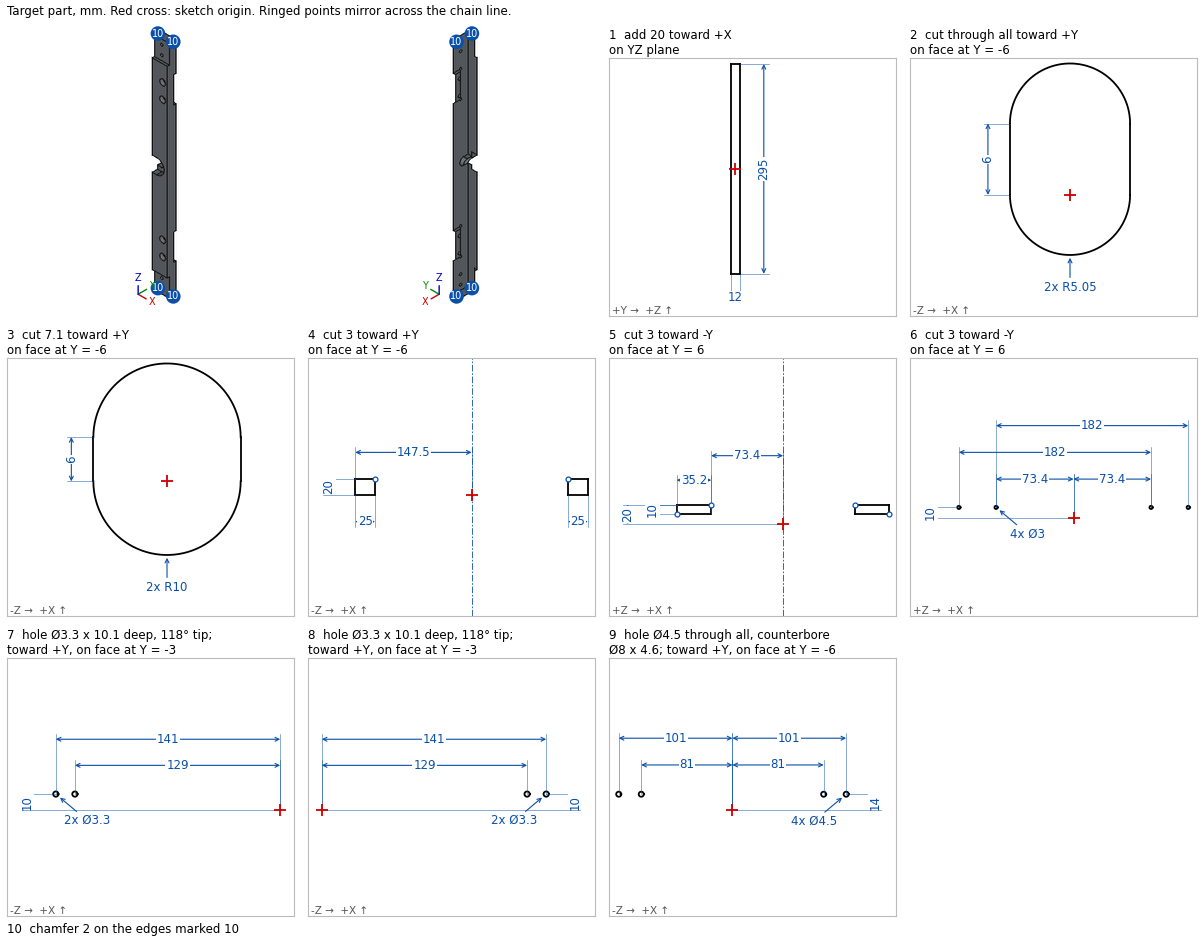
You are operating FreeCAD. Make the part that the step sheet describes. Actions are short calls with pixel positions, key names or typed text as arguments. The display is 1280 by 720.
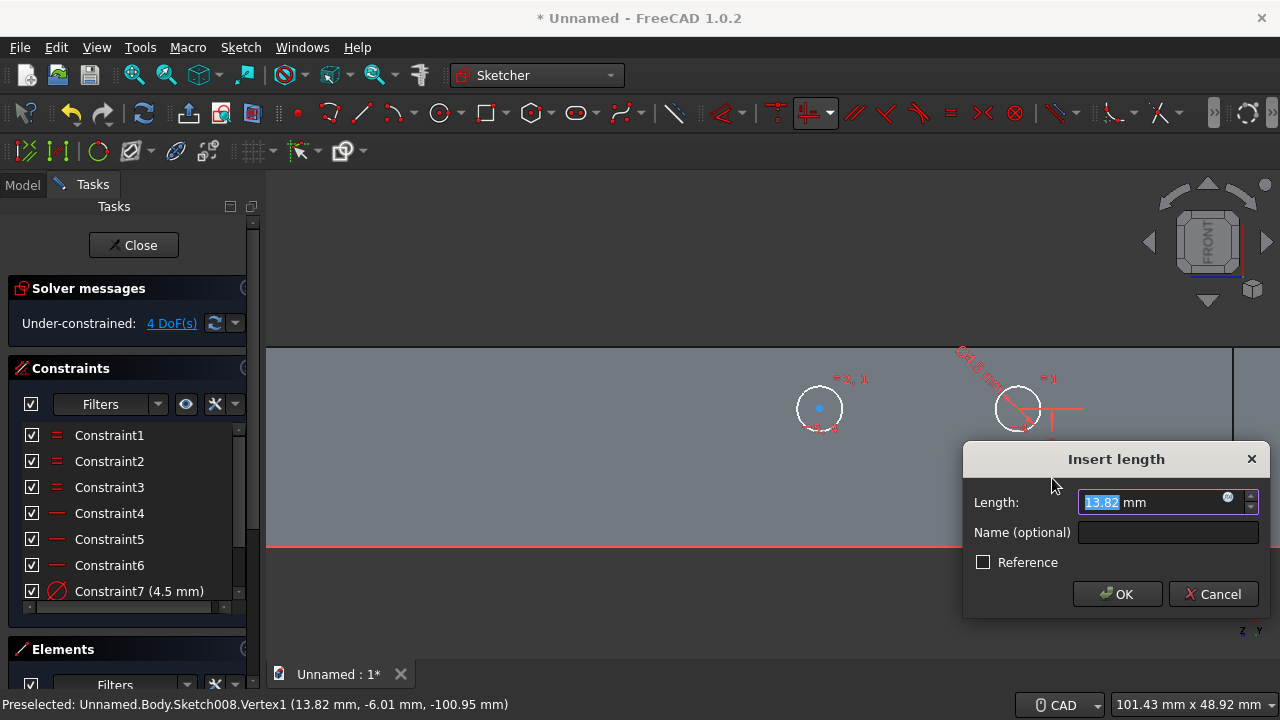
text(14)
key(Return)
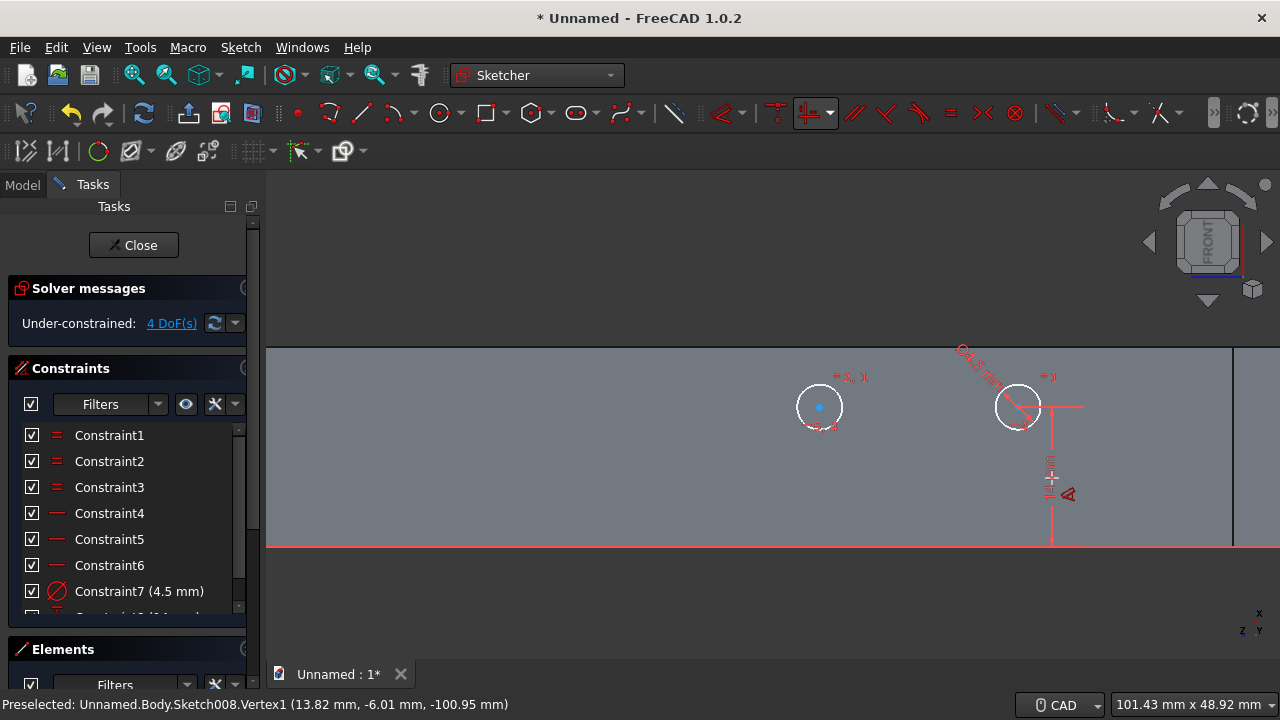
click(820, 407)
click(557, 581)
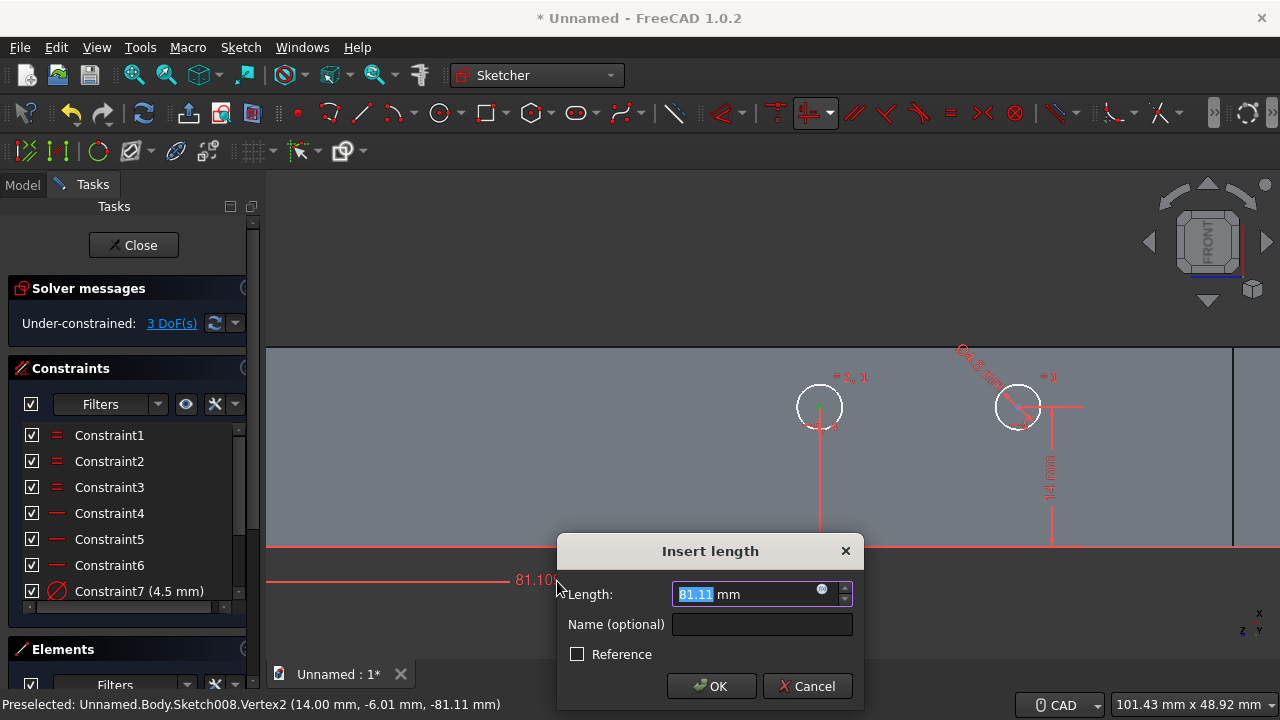
text(81)
key(Return)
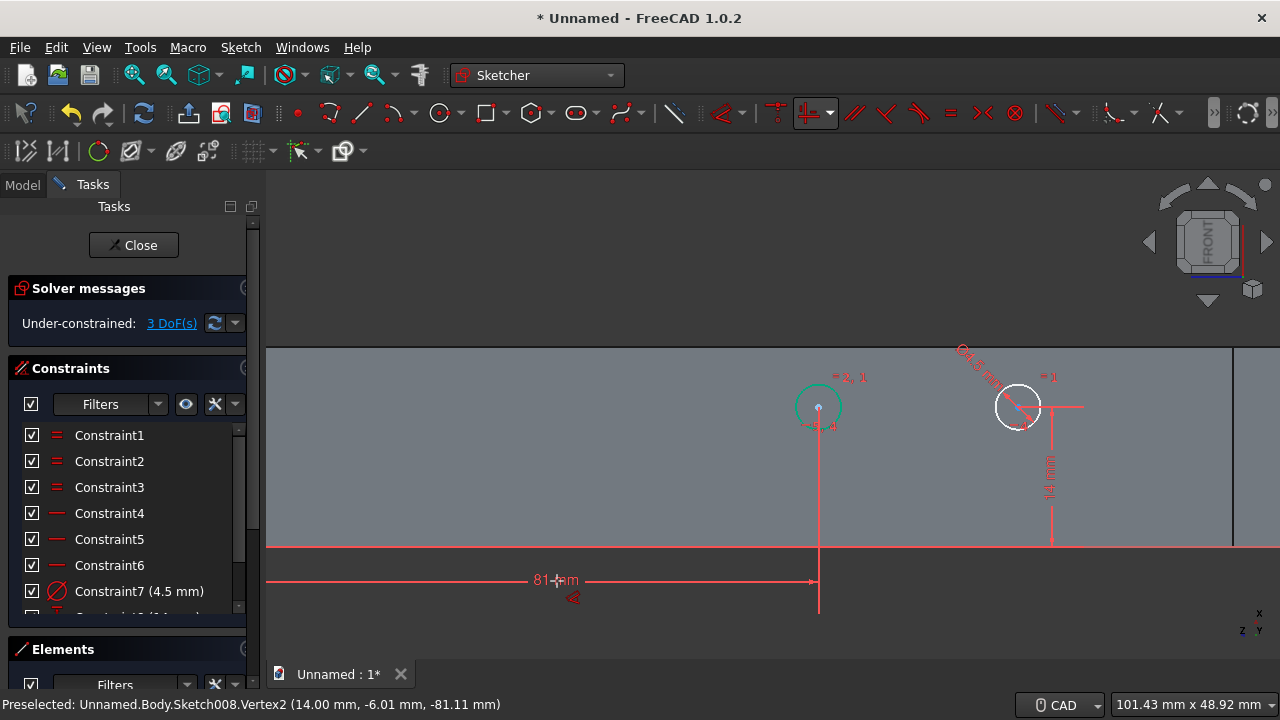
scroll(1004, 392, down, 6)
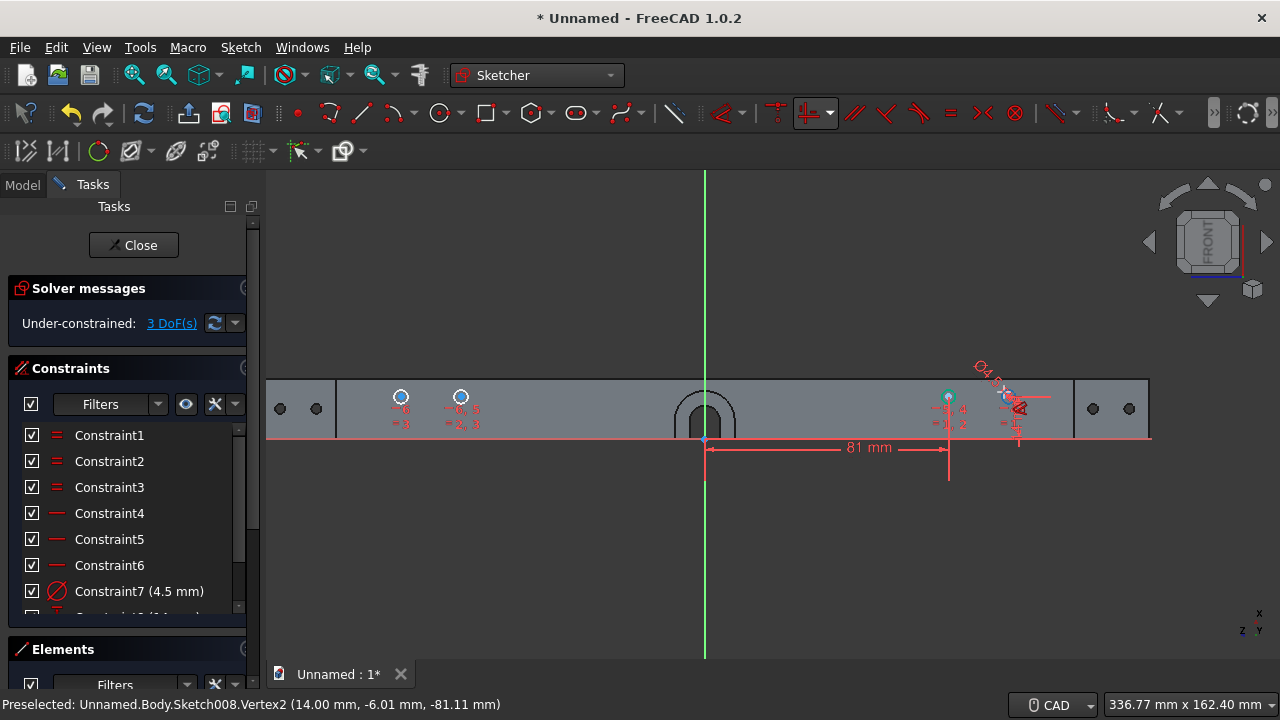
click(461, 397)
click(583, 473)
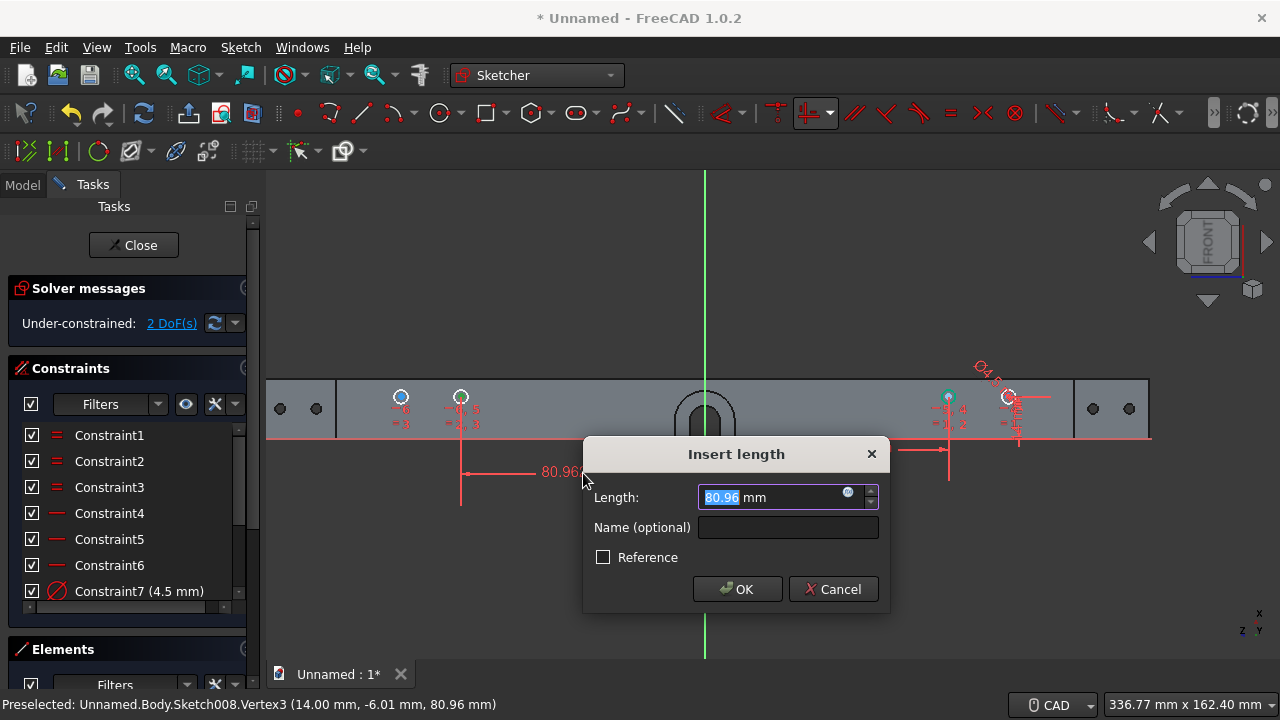
text(81)
key(Return)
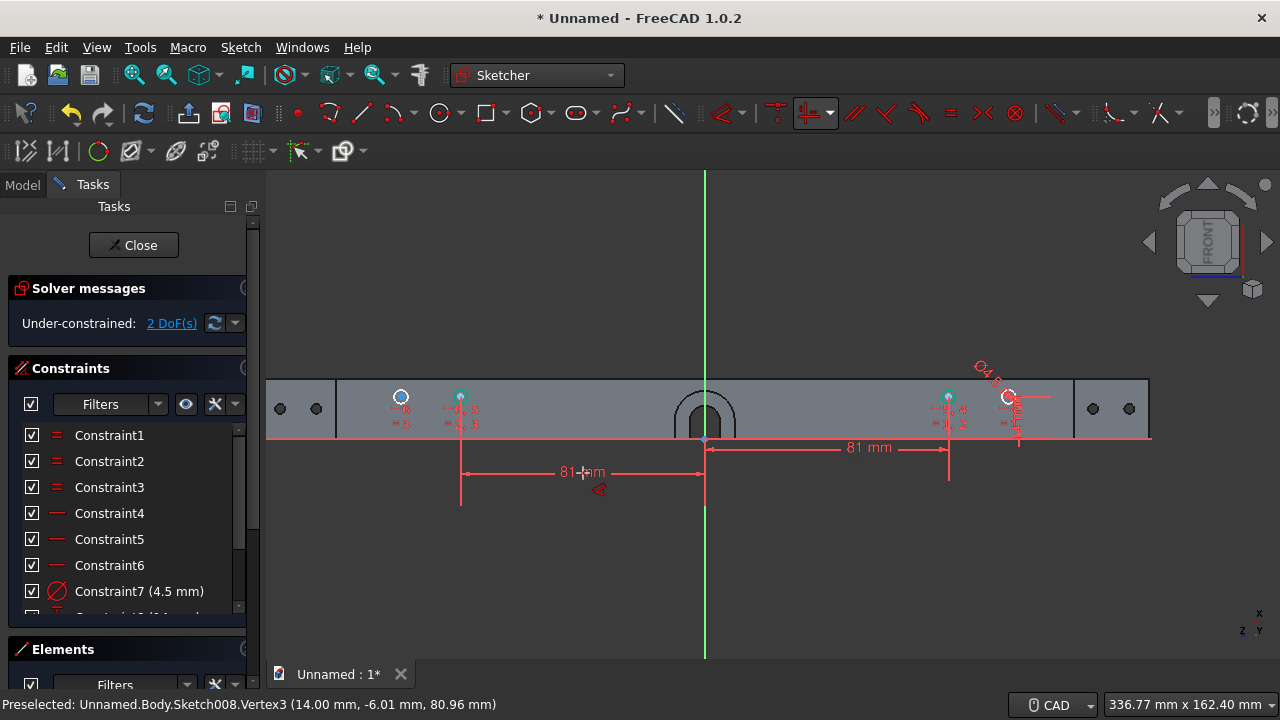
click(1009, 397)
click(857, 473)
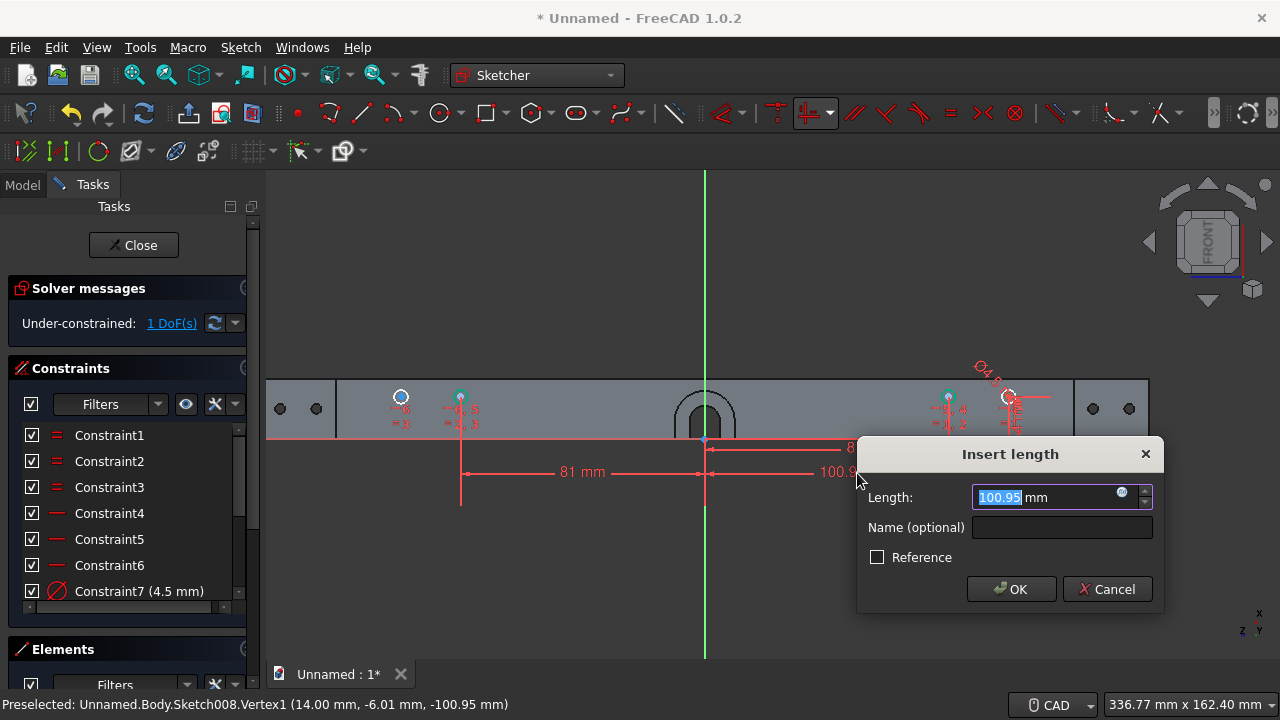
text(101)
key(Return)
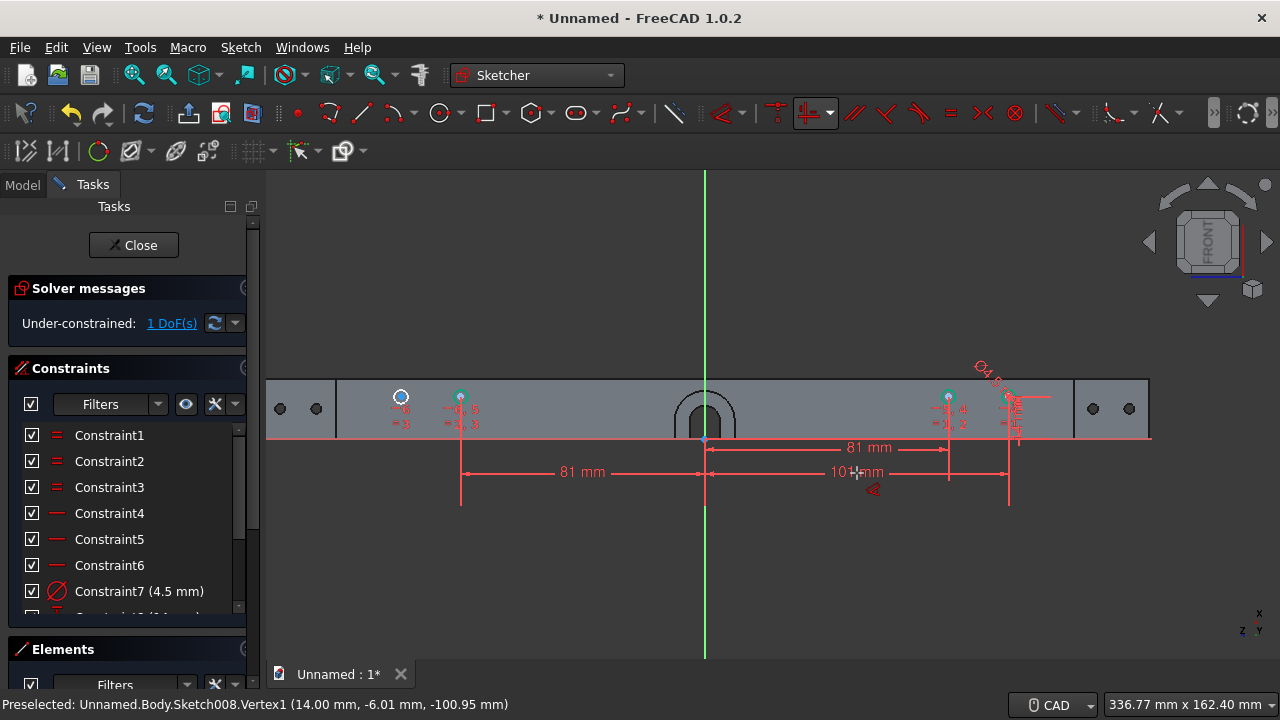
click(401, 397)
click(483, 473)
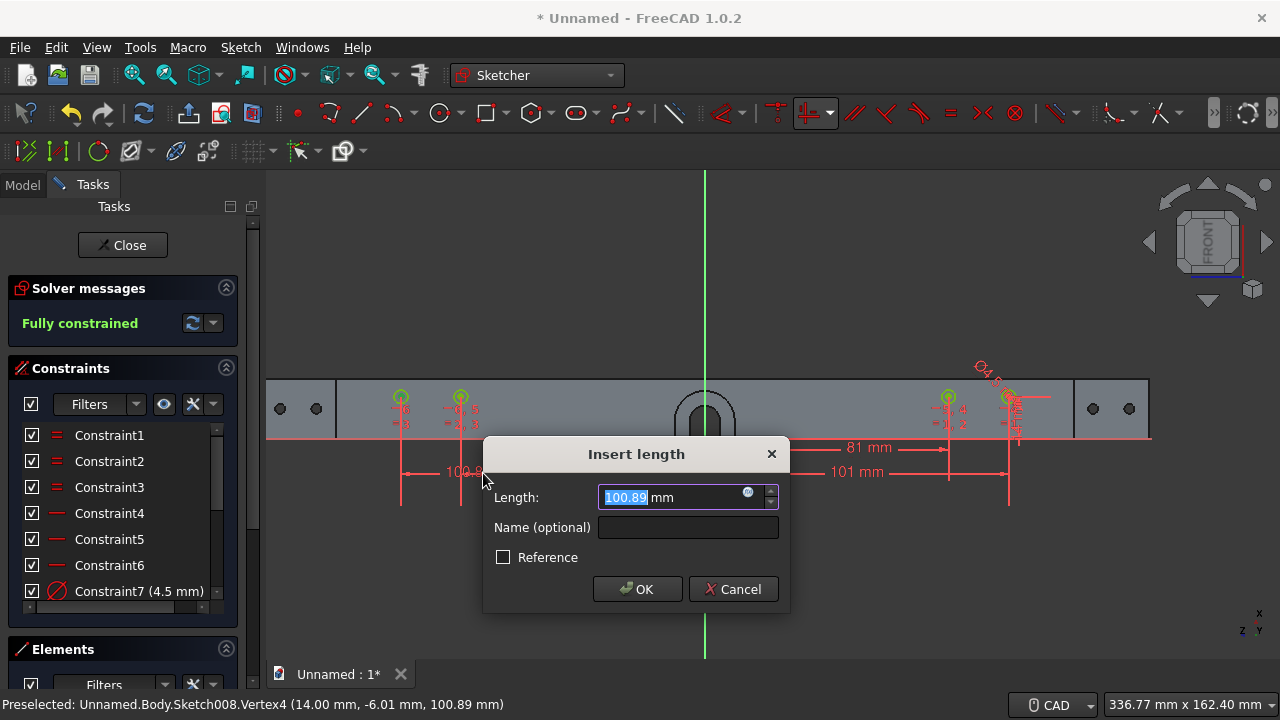
text(101)
key(Return)
key(Escape)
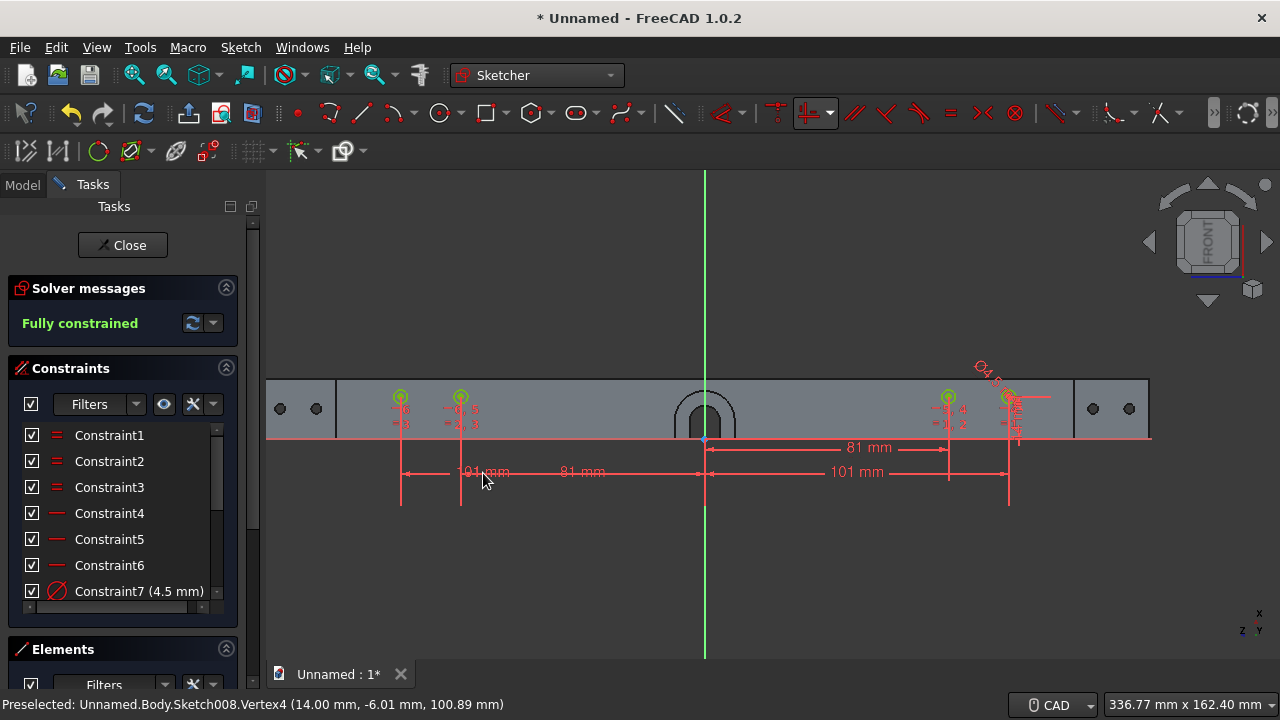
click(123, 245)